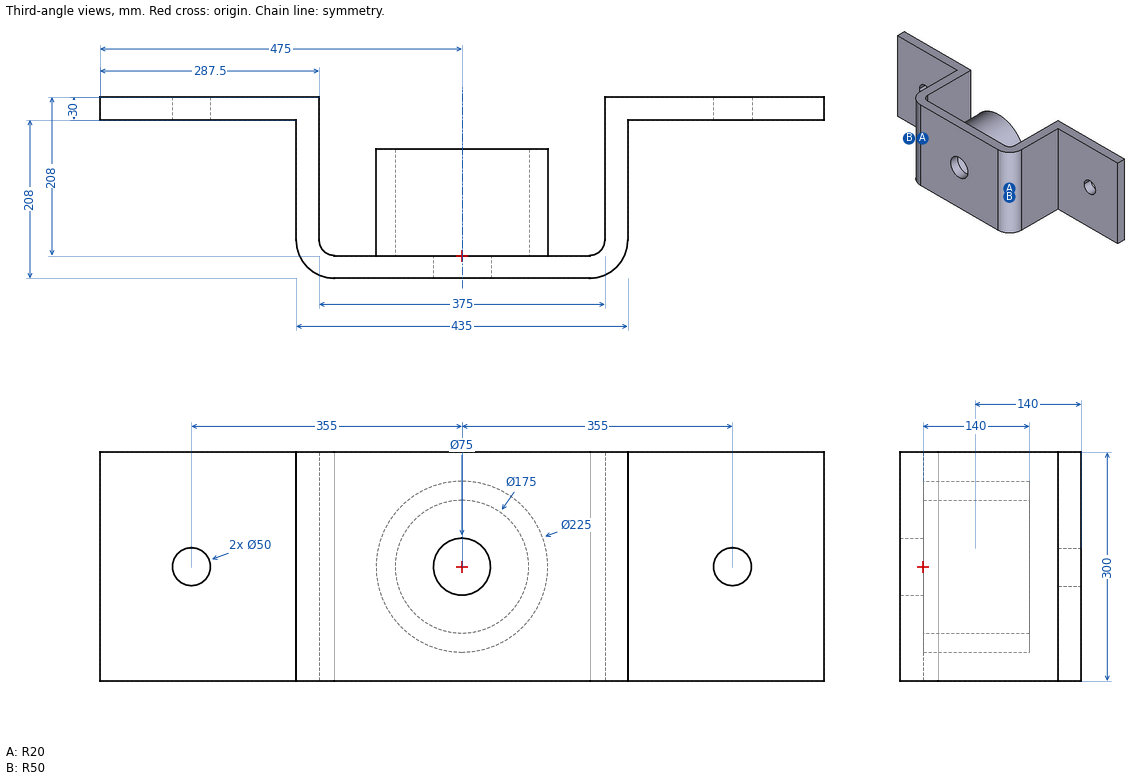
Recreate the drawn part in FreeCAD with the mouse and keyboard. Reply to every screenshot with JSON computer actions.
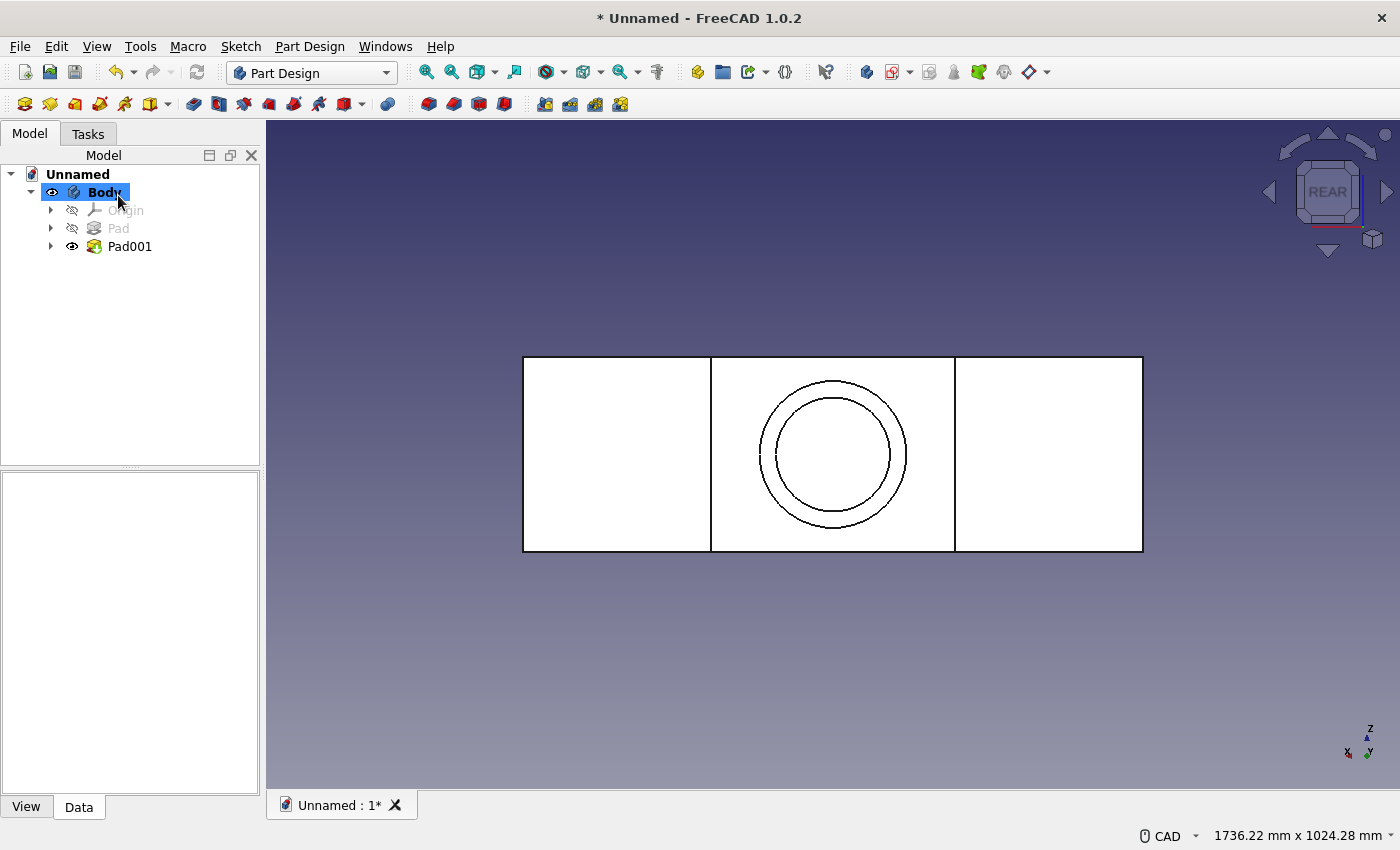
{"action": "left_click", "coordinate": [892, 72]}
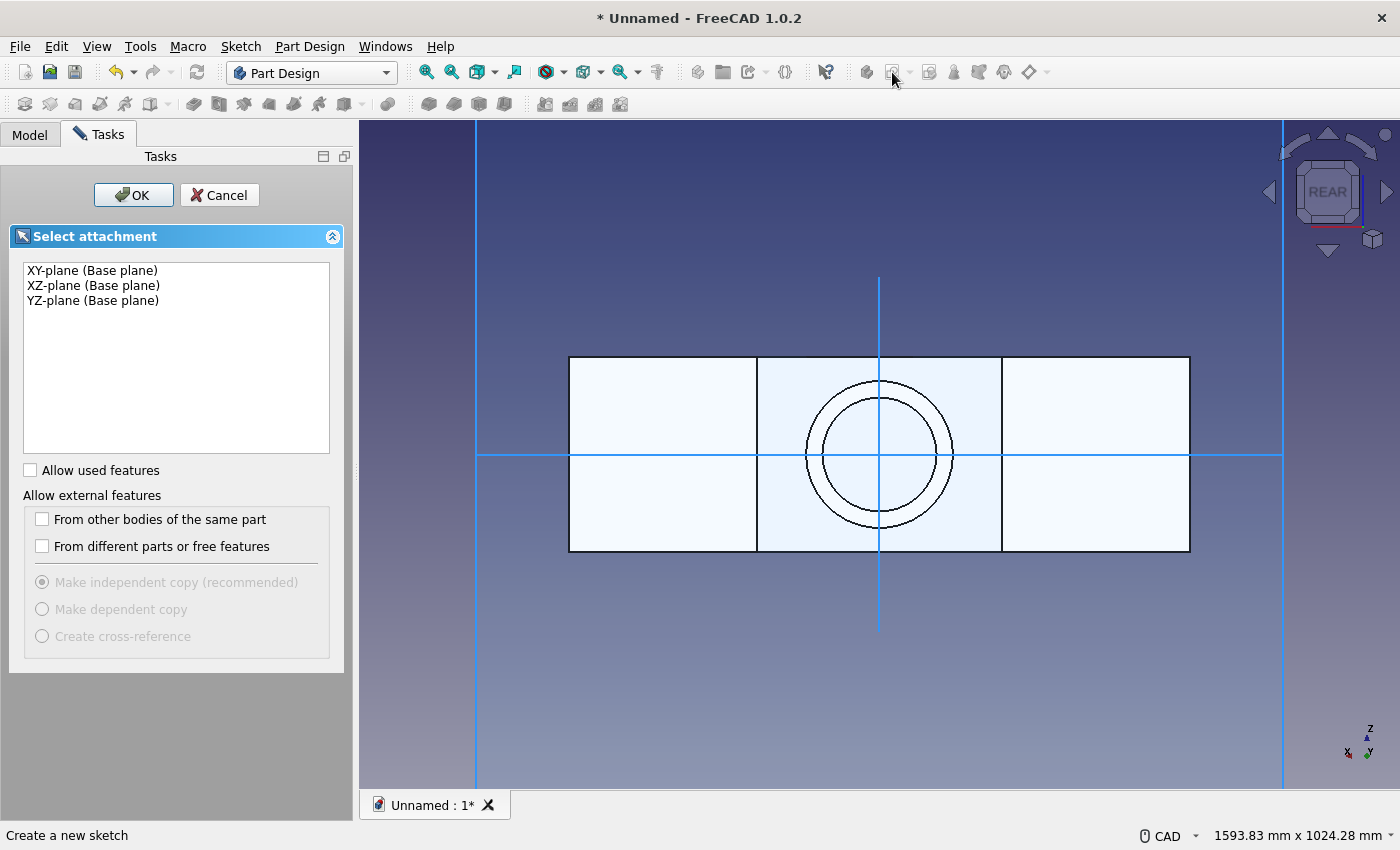
{"action": "left_click", "coordinate": [84, 286]}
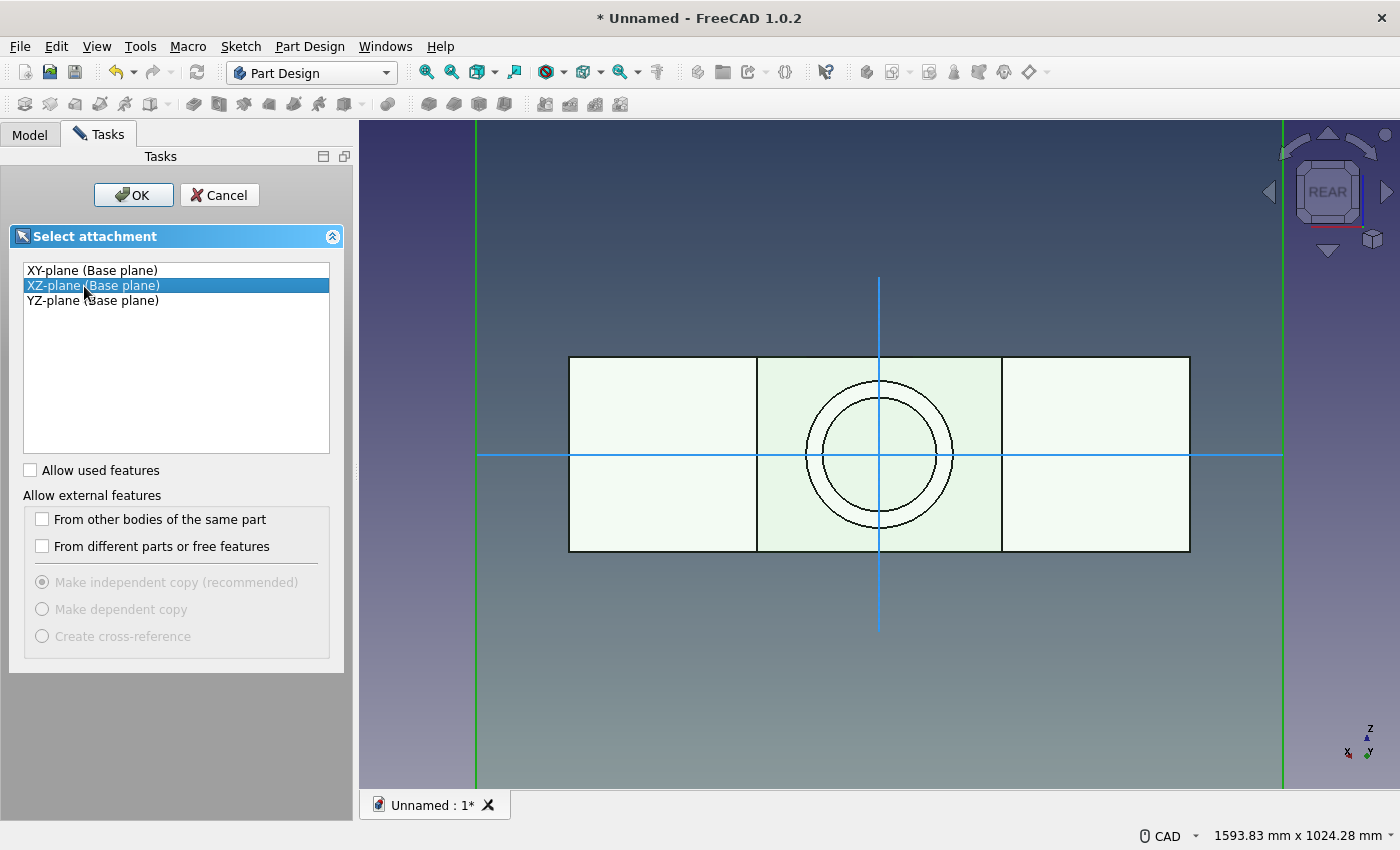
{"action": "left_click", "coordinate": [134, 195]}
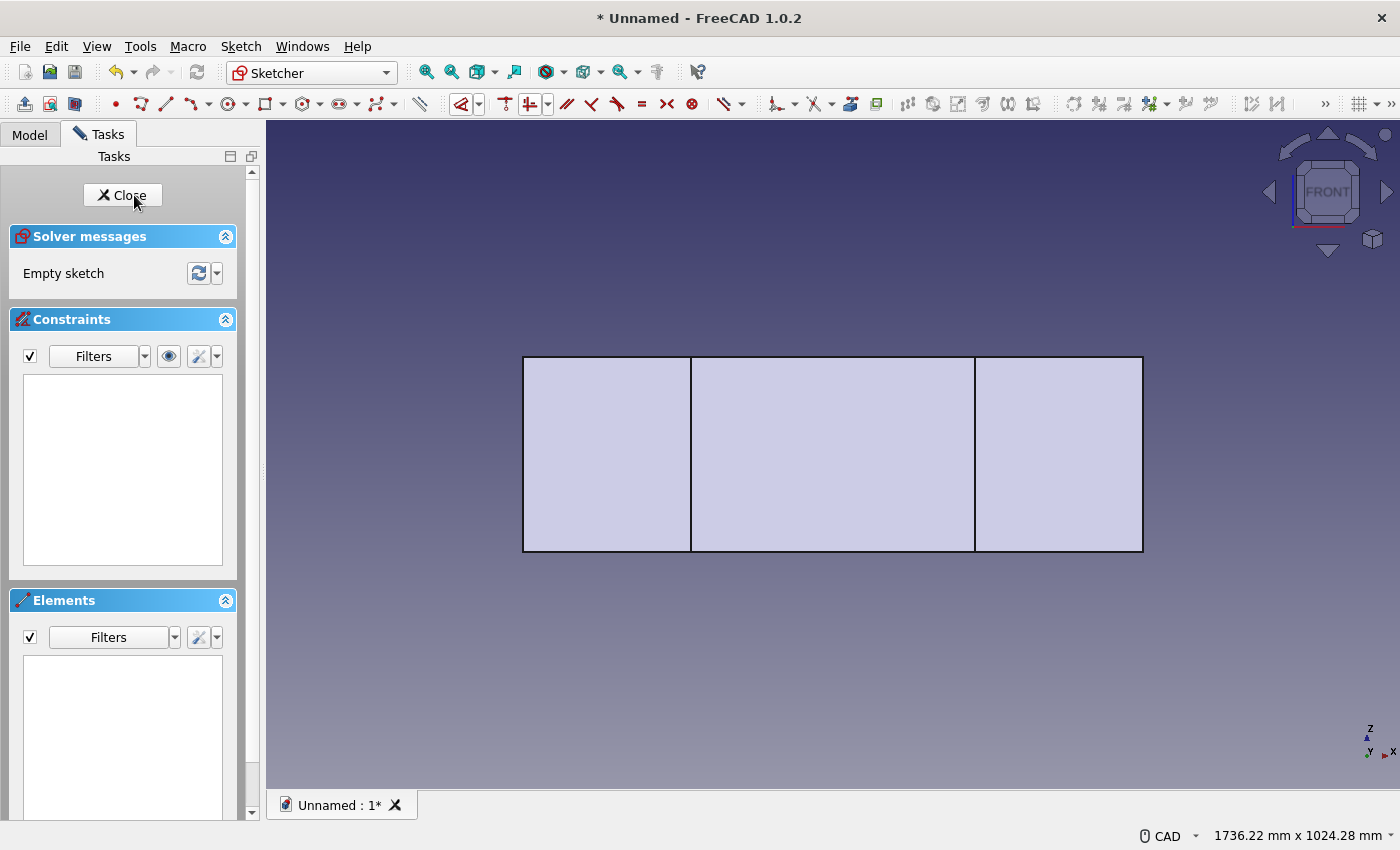
{"action": "left_click", "coordinate": [75, 104]}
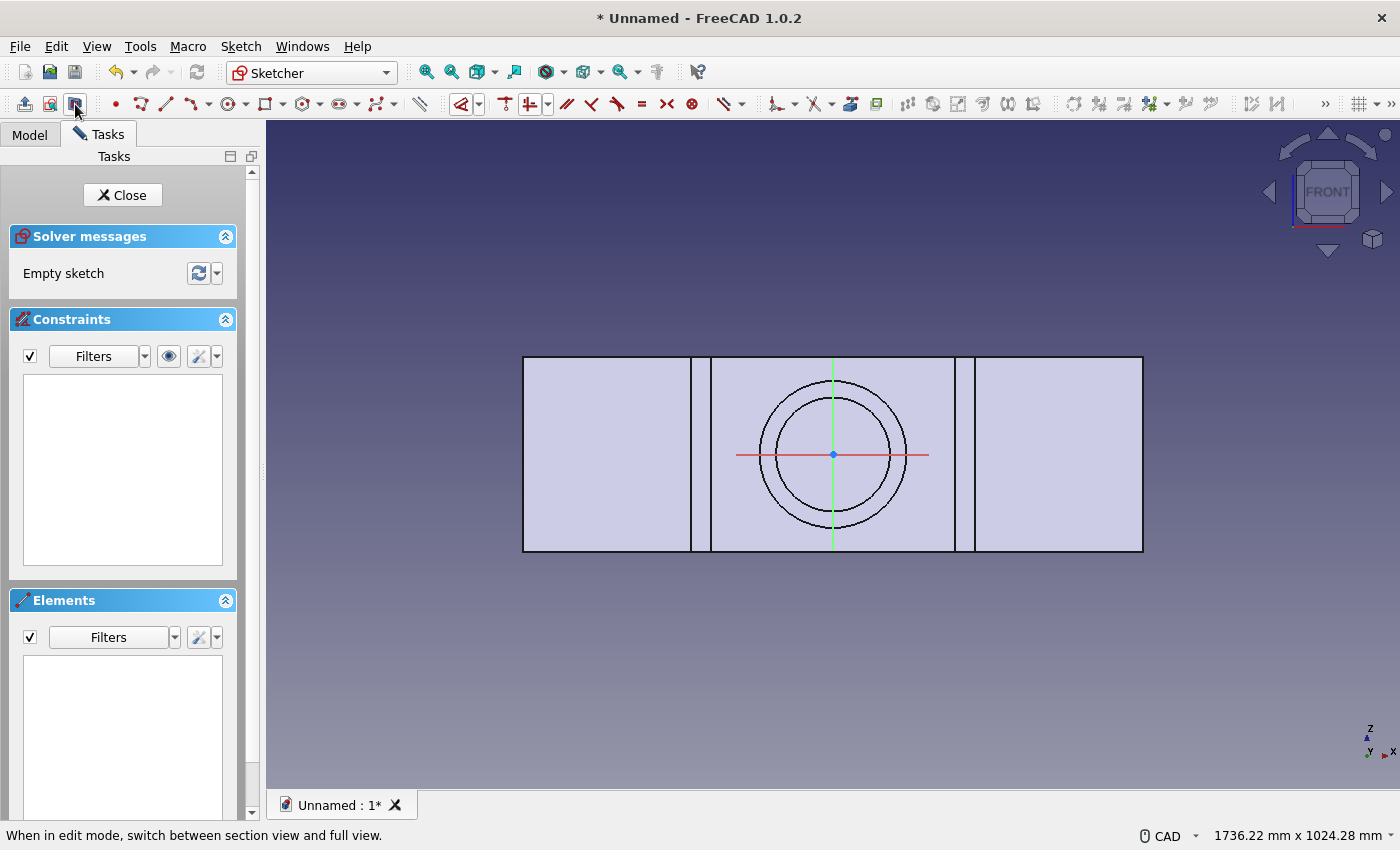
{"action": "scroll", "coordinate": [842, 455], "scroll_direction": "up", "scroll_amount": 11}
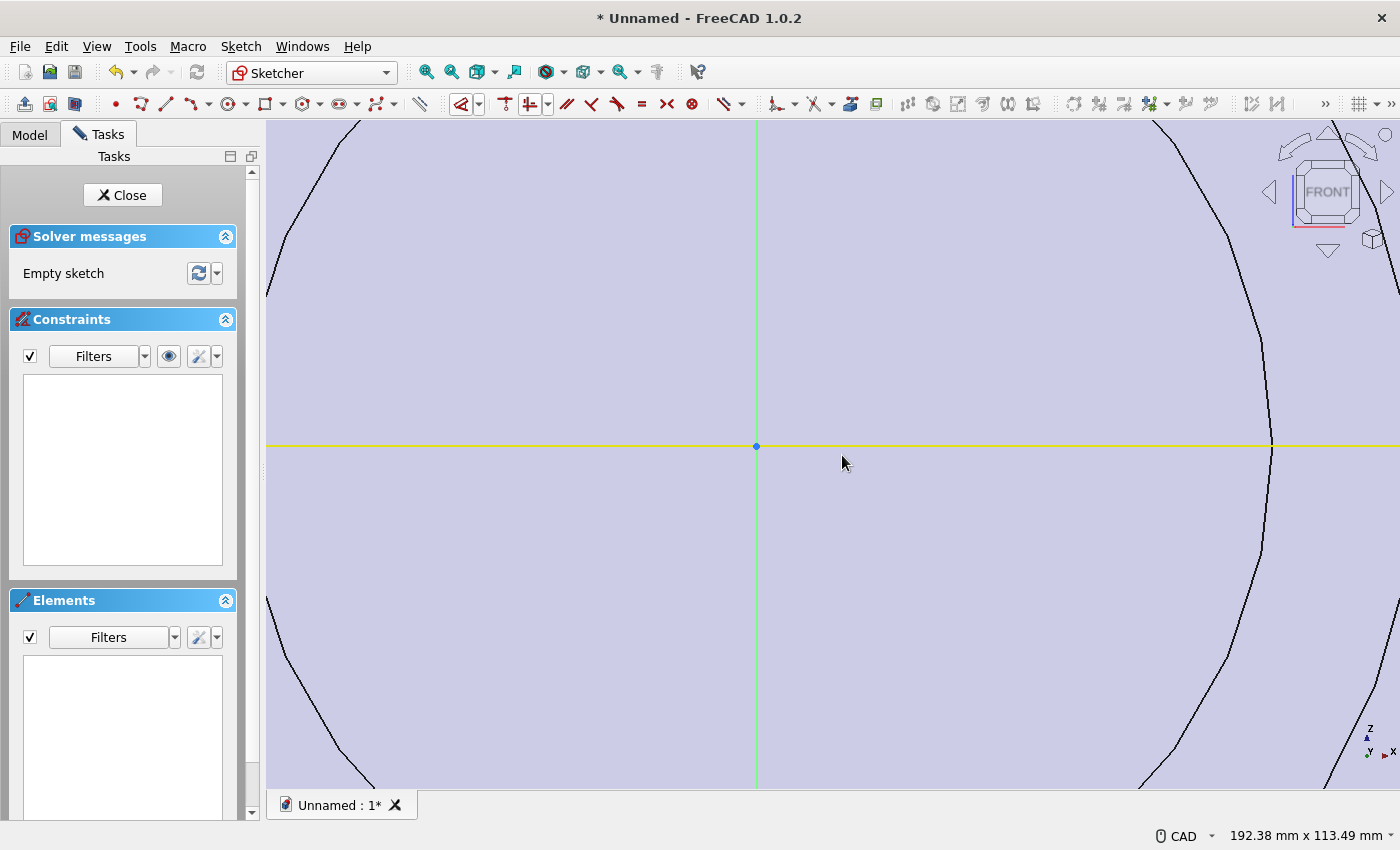
{"action": "left_click", "coordinate": [228, 104]}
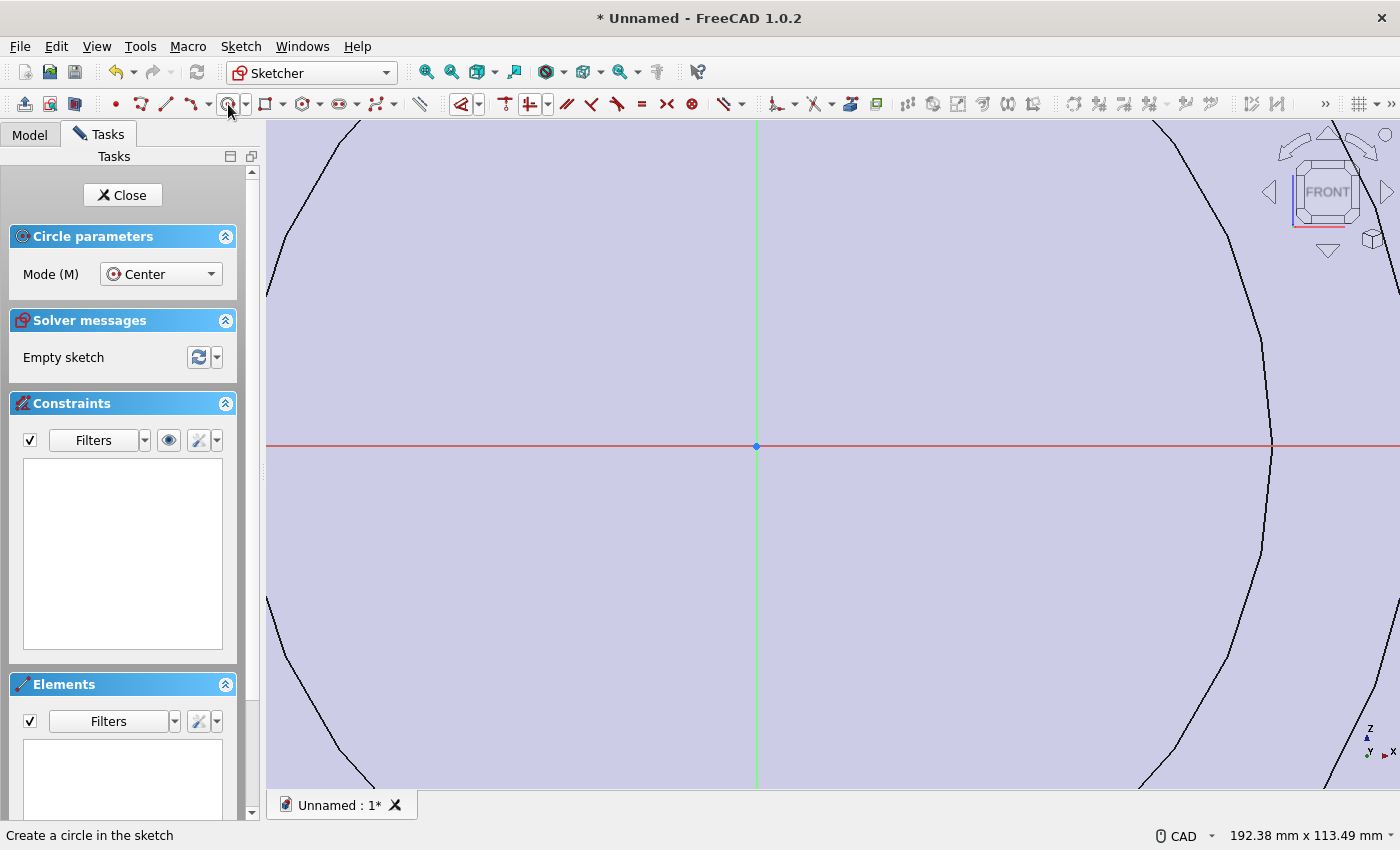
{"action": "left_click", "coordinate": [757, 446]}
{"action": "mouse_move", "coordinate": [913, 290]}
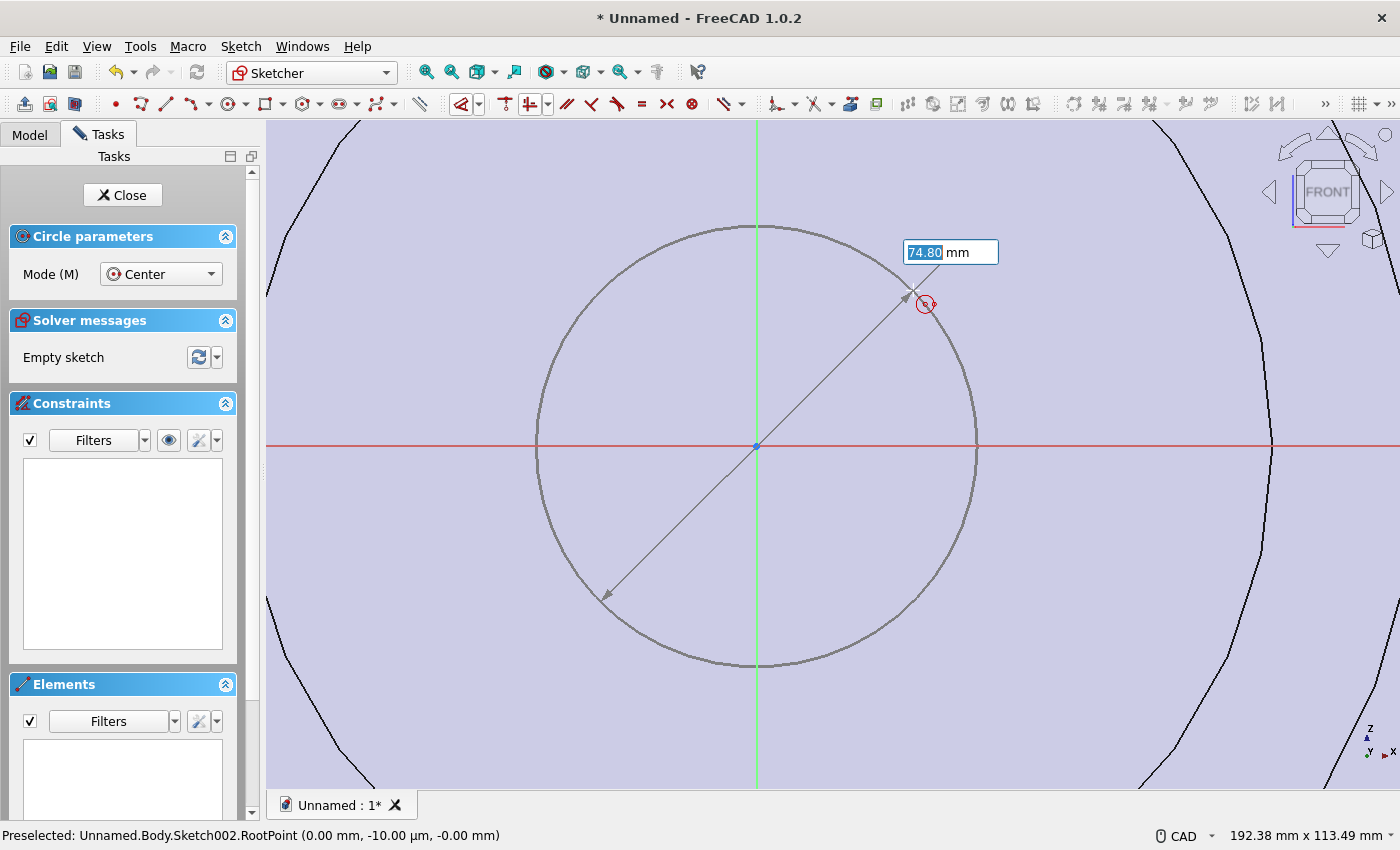
{"action": "type", "text": "75"}
{"action": "key", "text": "Return"}
{"action": "key", "text": "Escape"}